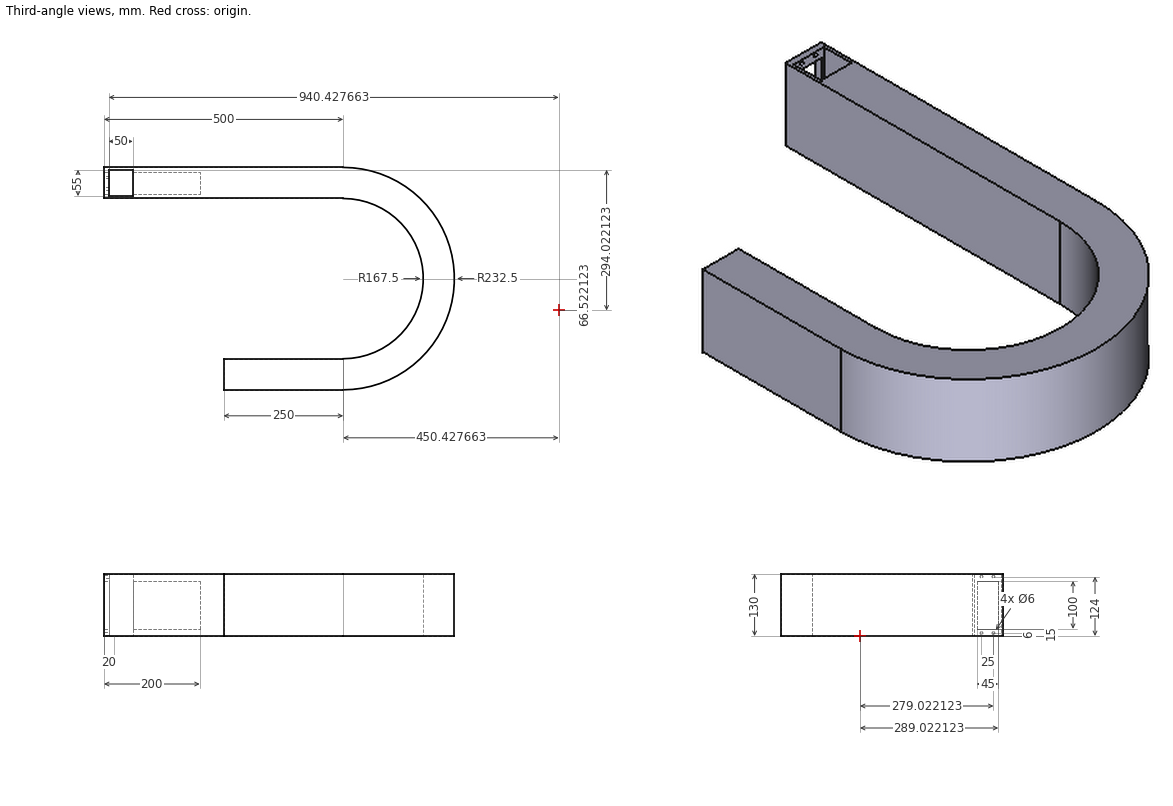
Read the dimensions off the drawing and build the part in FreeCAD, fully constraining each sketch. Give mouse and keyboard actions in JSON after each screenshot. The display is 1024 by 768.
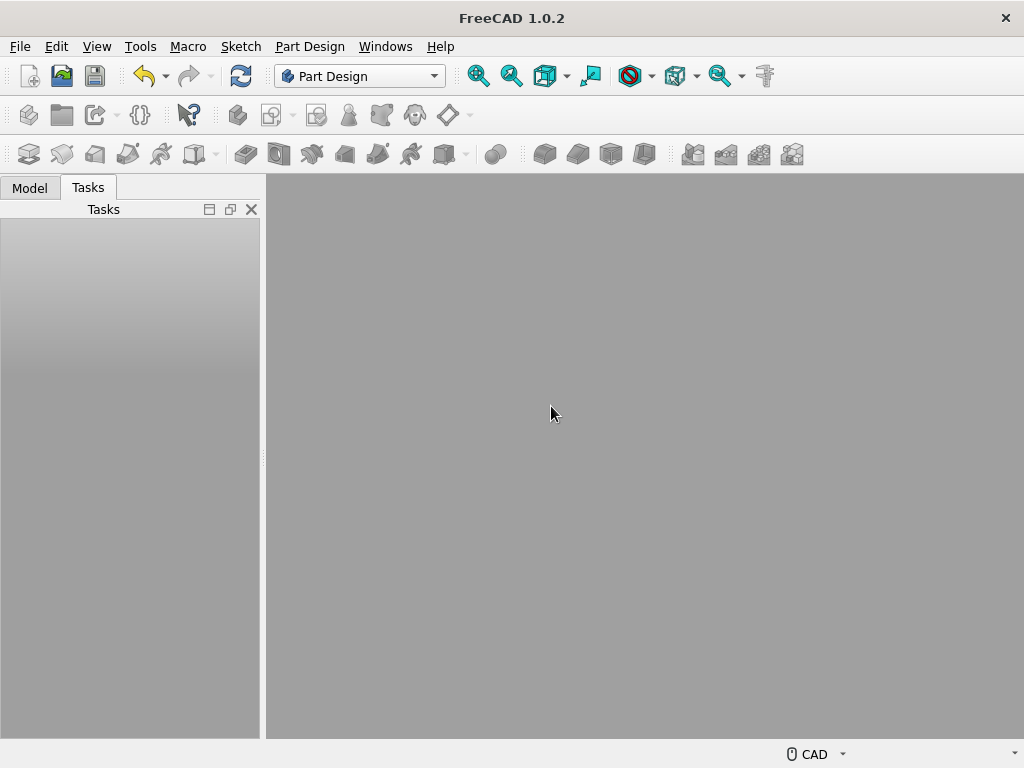
{"action": "key", "text": "ctrl+n"}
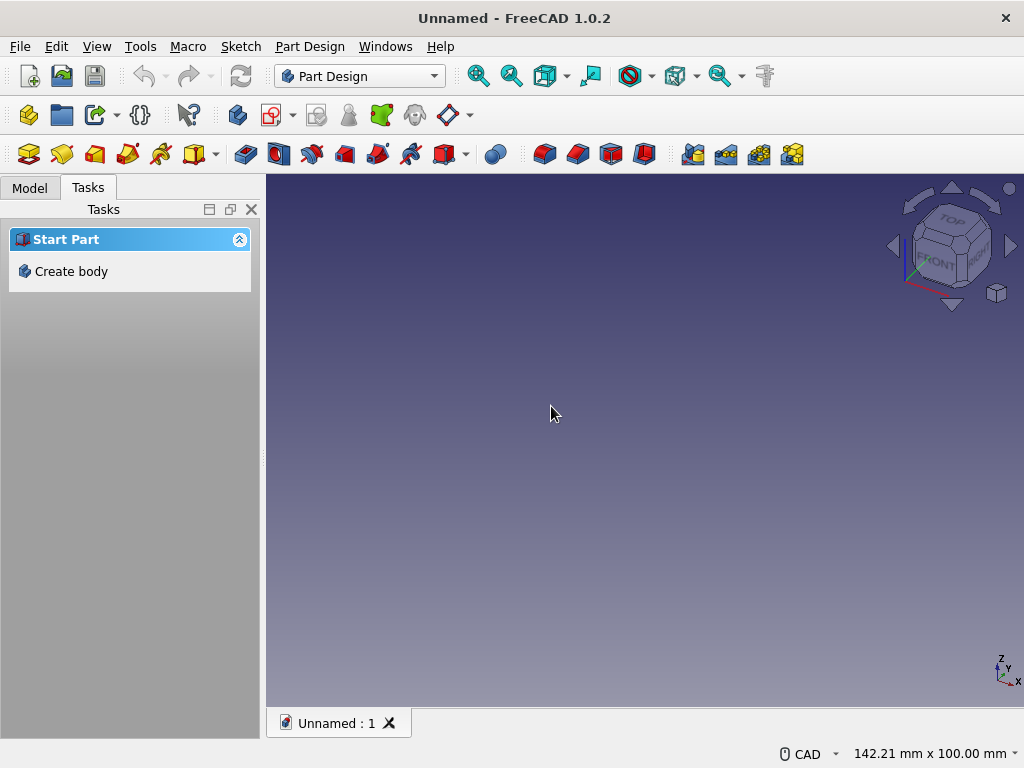
{"action": "left_click", "coordinate": [270, 116]}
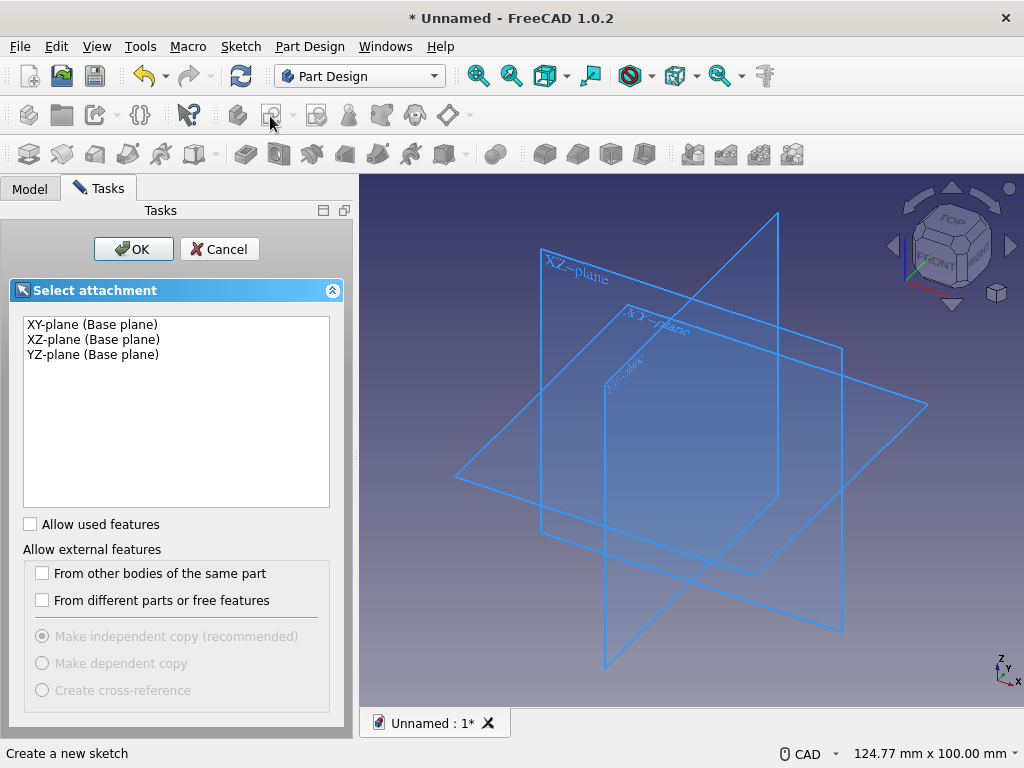
{"action": "left_click", "coordinate": [84, 324]}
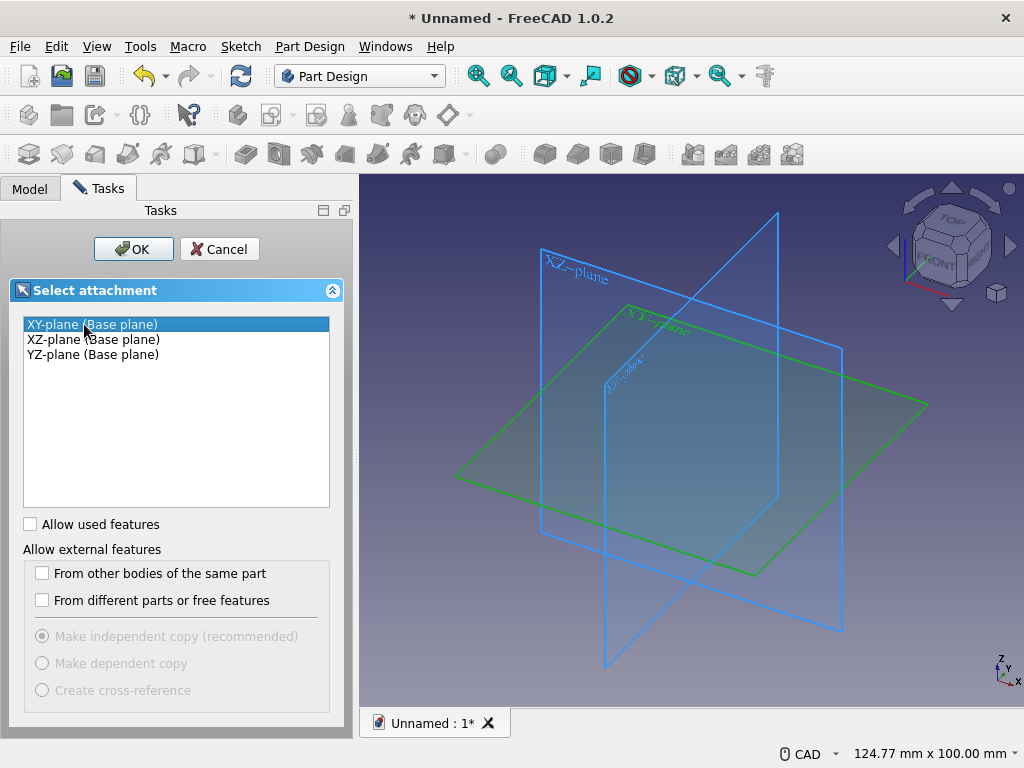
{"action": "left_click", "coordinate": [134, 249]}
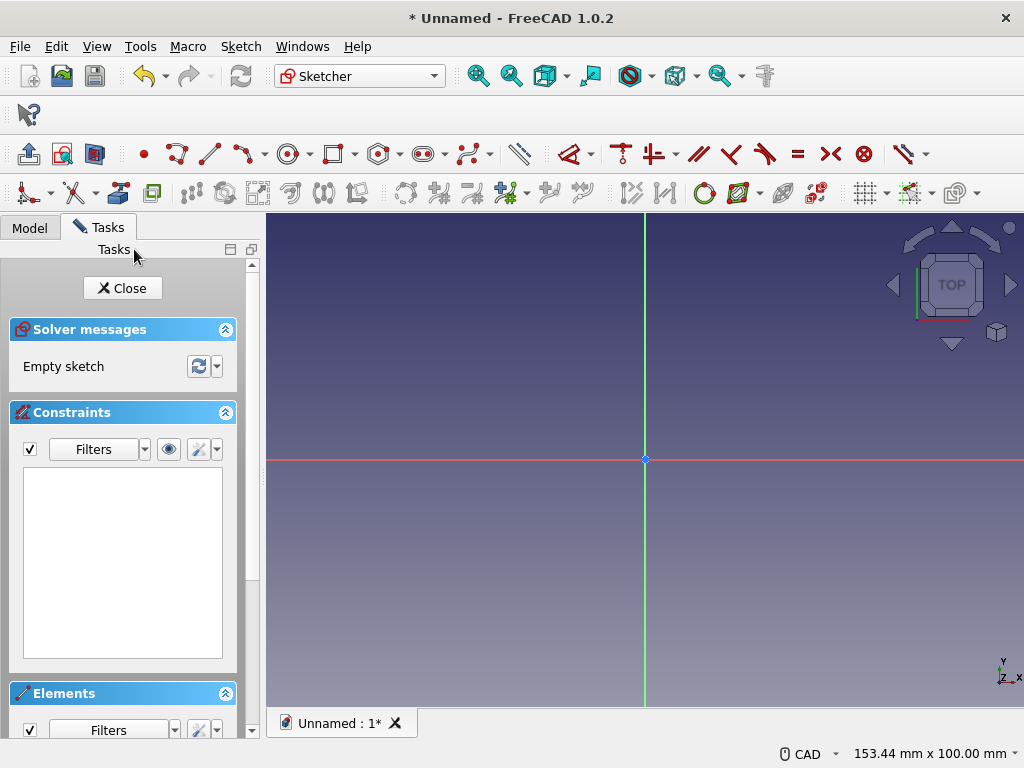
{"action": "scroll", "coordinate": [804, 493], "scroll_direction": "down", "scroll_amount": 12}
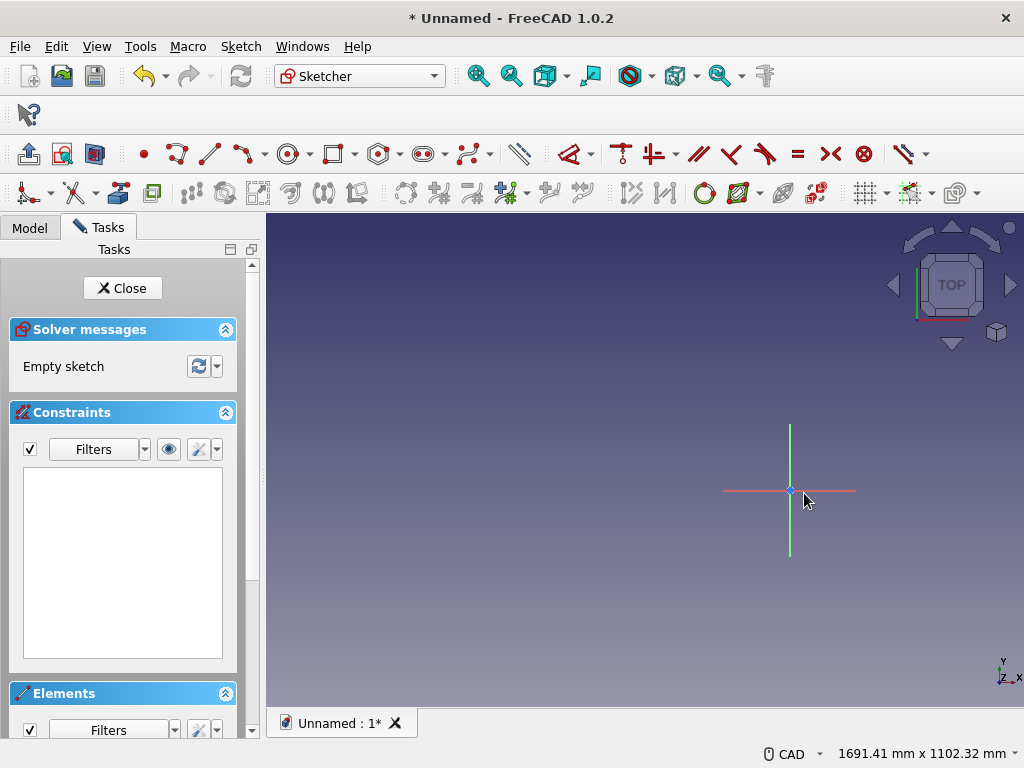
{"action": "key", "text": "g m"}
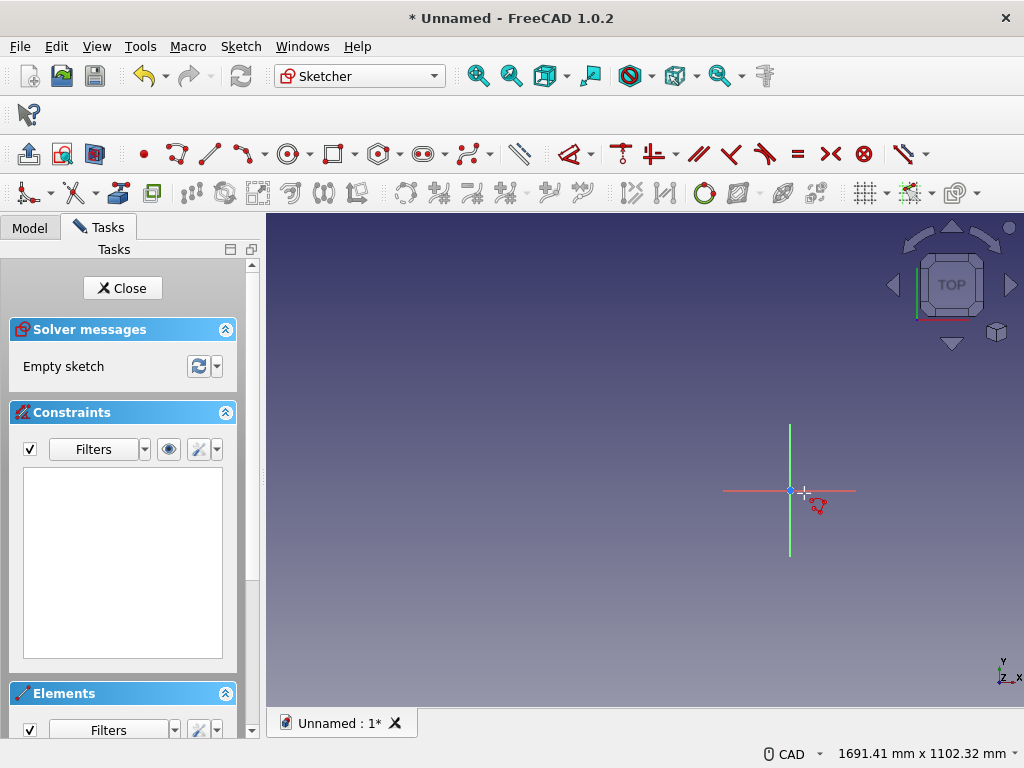
{"action": "left_click", "coordinate": [588, 536]}
{"action": "left_click", "coordinate": [476, 536]}
{"action": "left_click", "coordinate": [476, 565]}
{"action": "left_click", "coordinate": [588, 565]}
{"action": "right_click", "coordinate": [588, 565]}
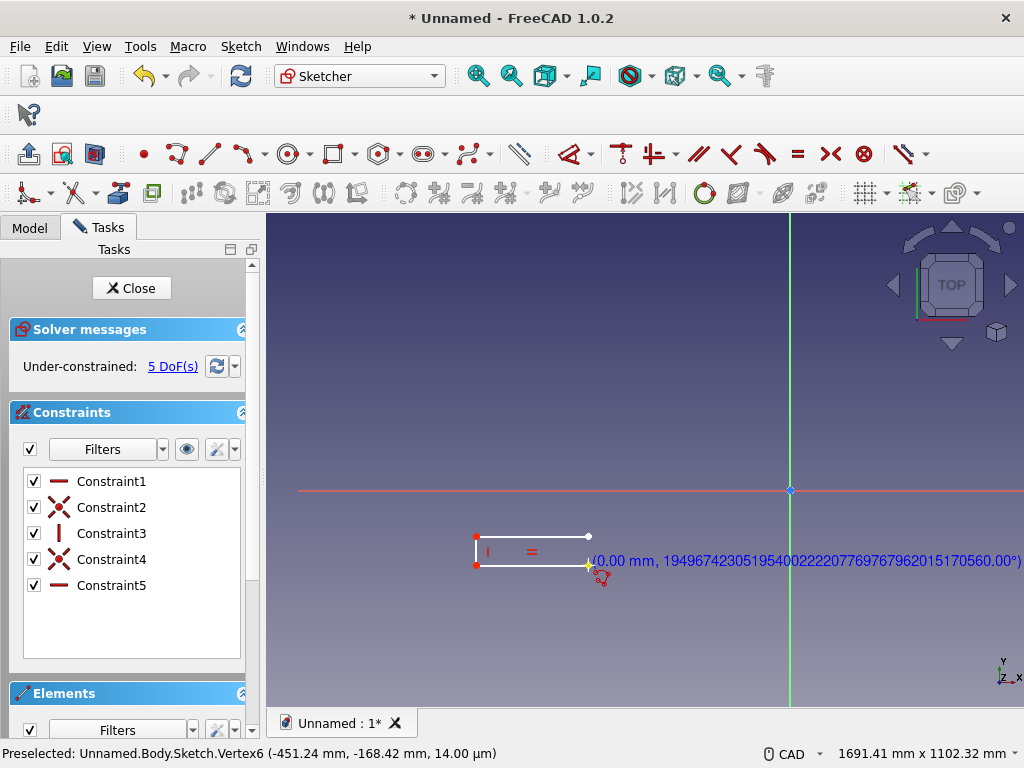
{"action": "left_click", "coordinate": [588, 357]}
{"action": "left_click", "coordinate": [364, 357]}
{"action": "left_click", "coordinate": [364, 386]}
{"action": "left_click", "coordinate": [588, 386]}
{"action": "right_click", "coordinate": [588, 386]}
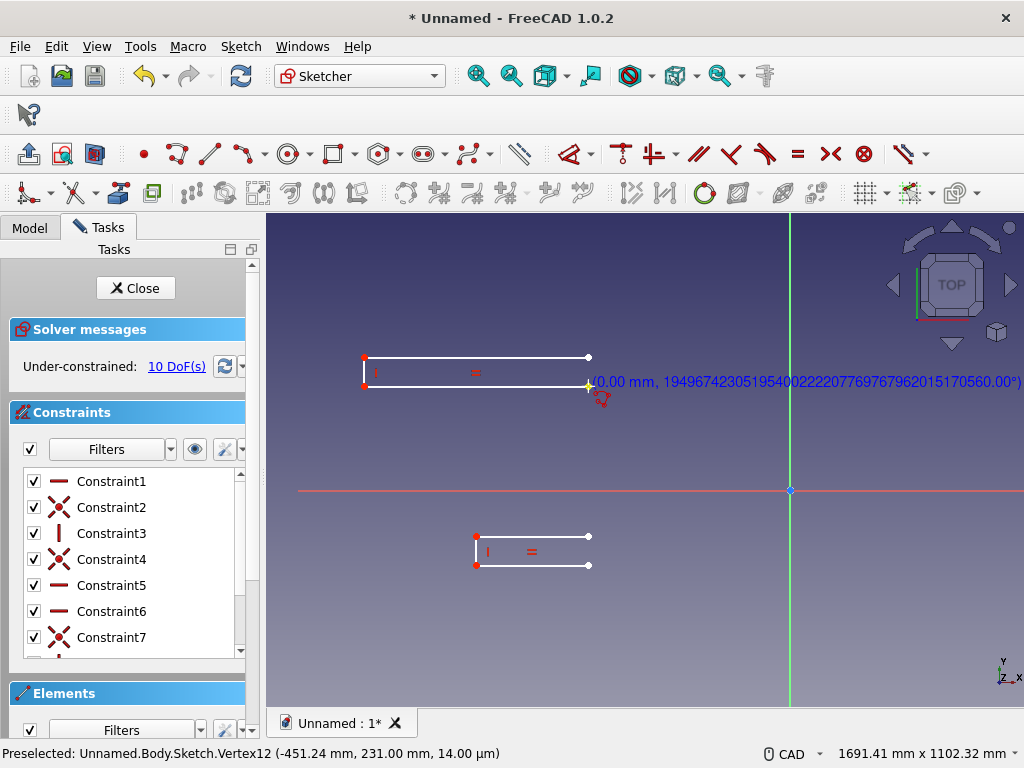
{"action": "key", "text": "g 3 a"}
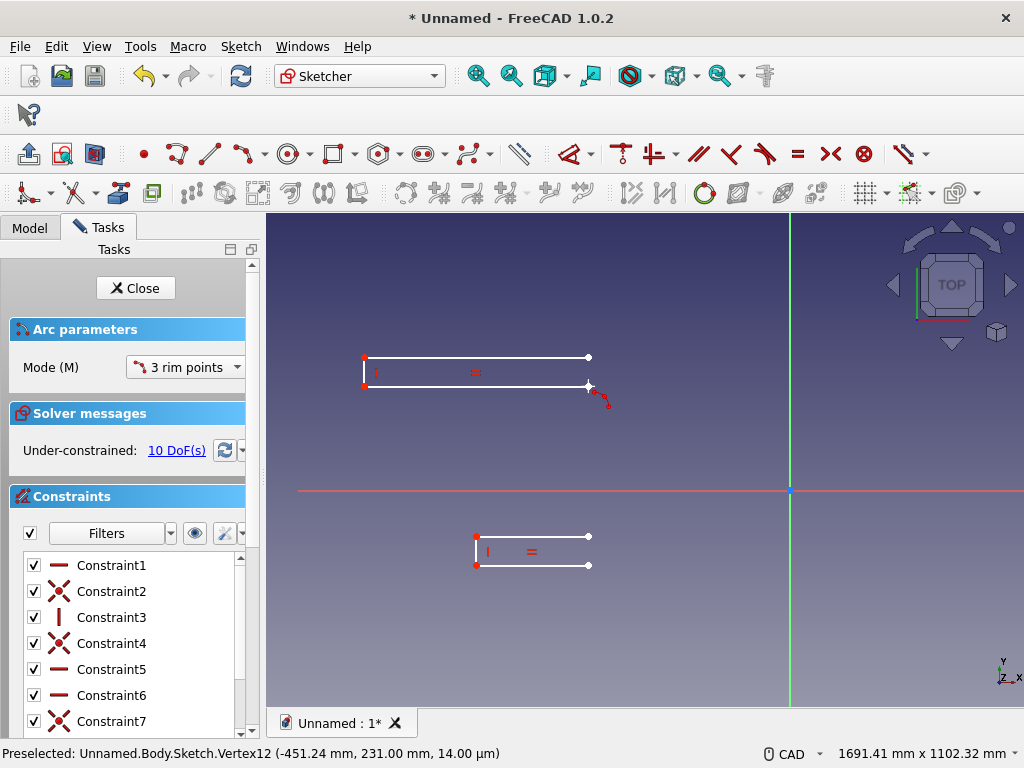
{"action": "left_click", "coordinate": [588, 566]}
{"action": "left_click", "coordinate": [588, 358]}
{"action": "left_click", "coordinate": [693, 461]}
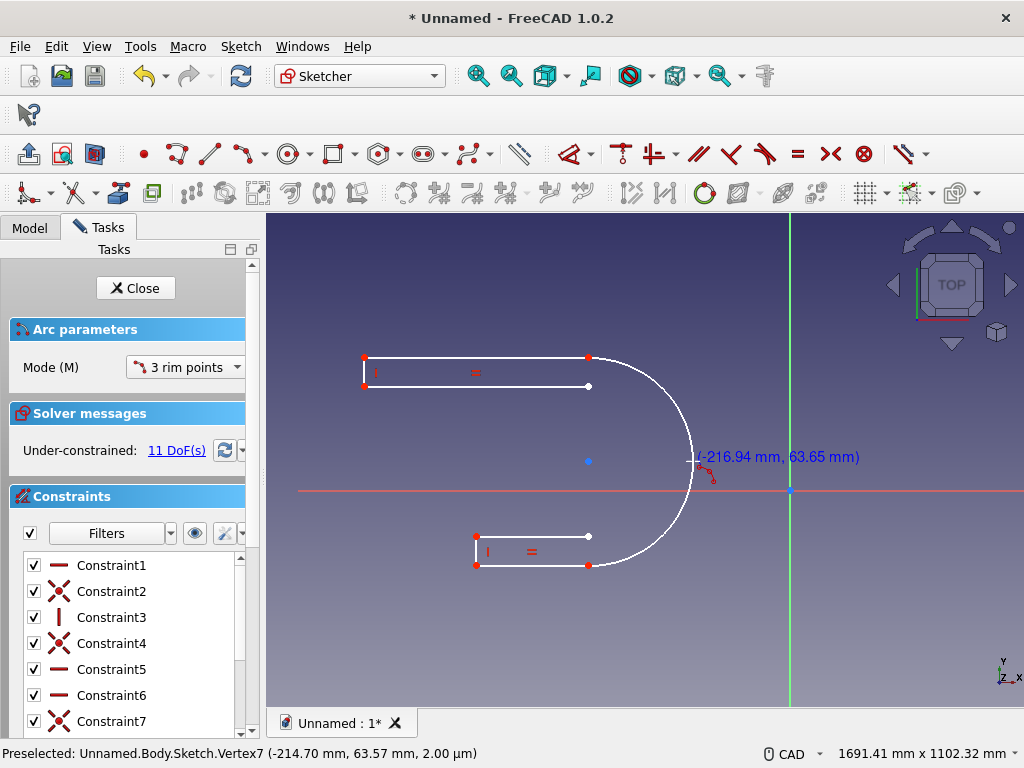
{"action": "left_click", "coordinate": [588, 387]}
{"action": "left_click", "coordinate": [588, 537]}
{"action": "left_click", "coordinate": [663, 461]}
{"action": "key", "text": "Escape"}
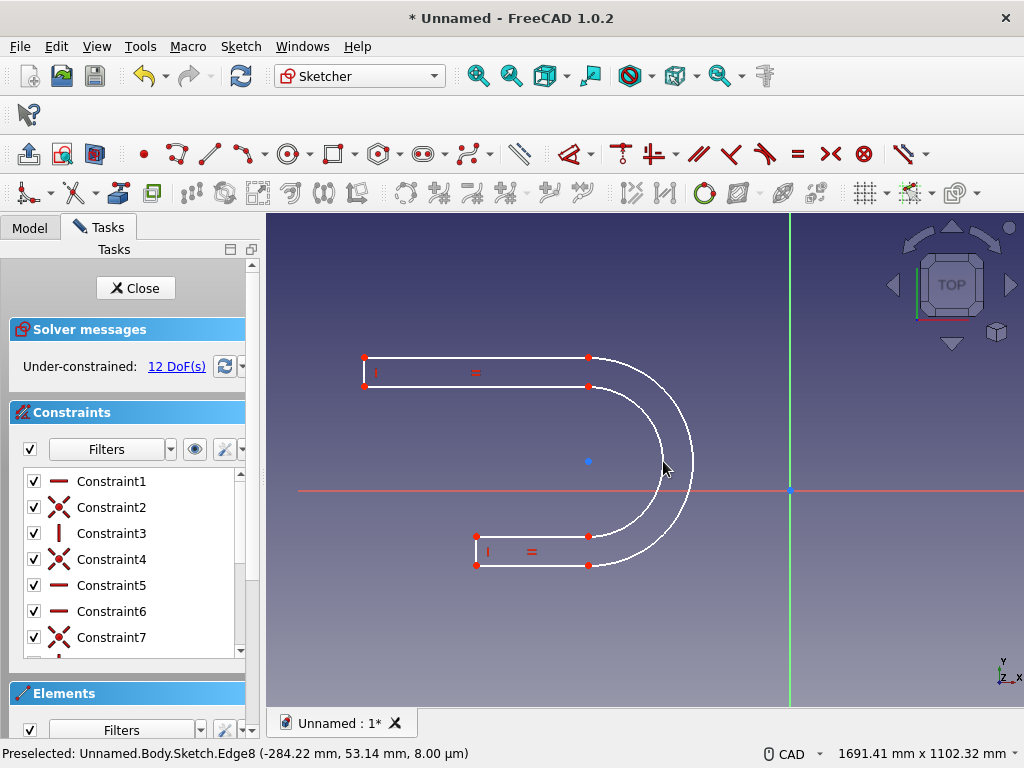
{"action": "left_click", "coordinate": [673, 523]}